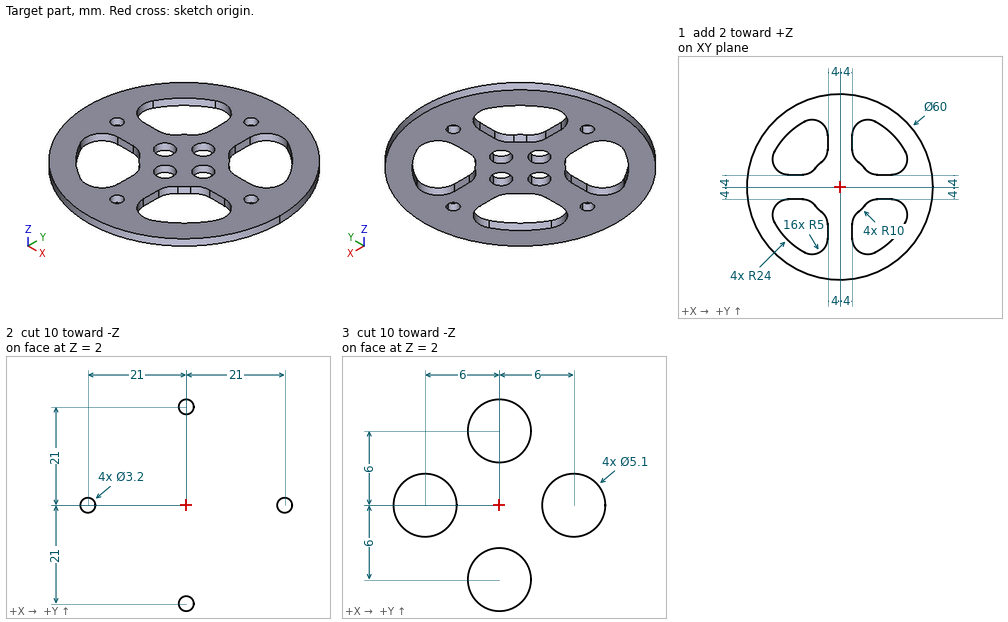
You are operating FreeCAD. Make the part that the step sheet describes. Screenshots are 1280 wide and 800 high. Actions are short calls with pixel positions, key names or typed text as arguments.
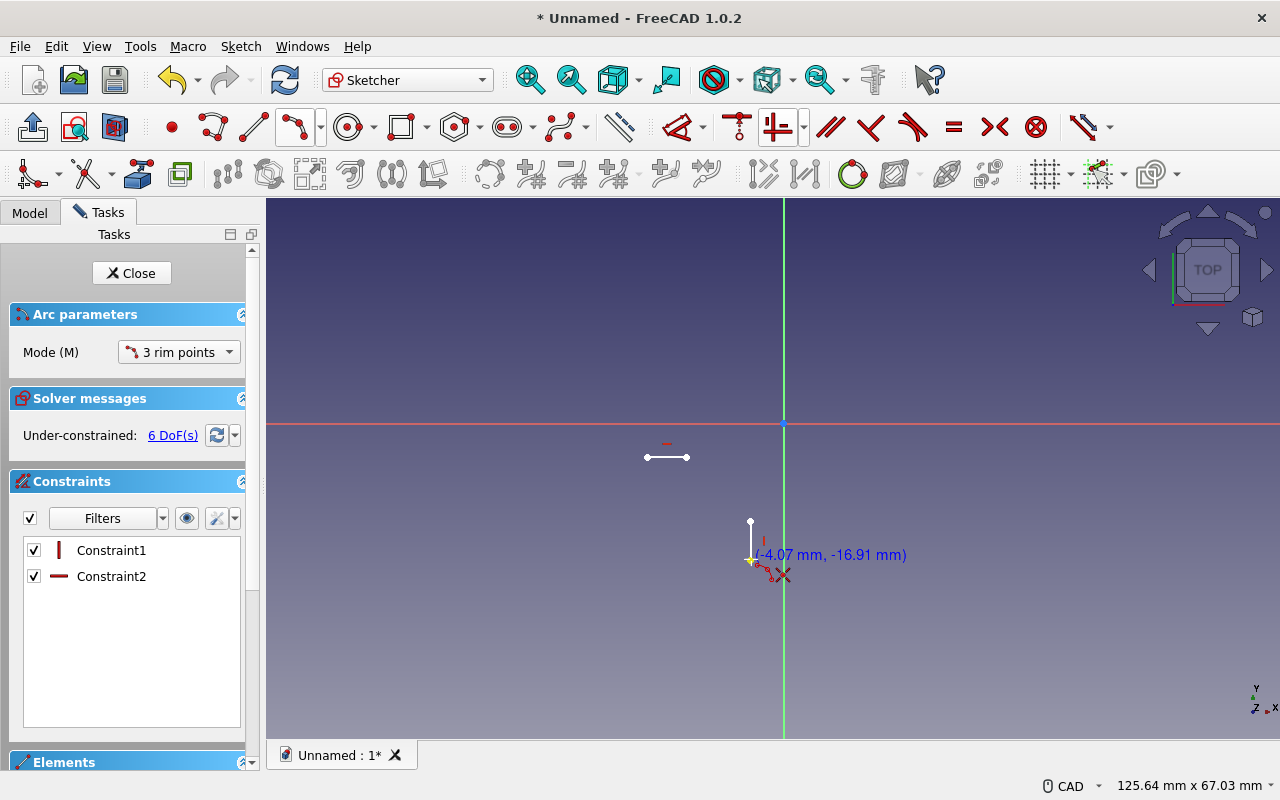
click(751, 560)
click(692, 594)
click(732, 593)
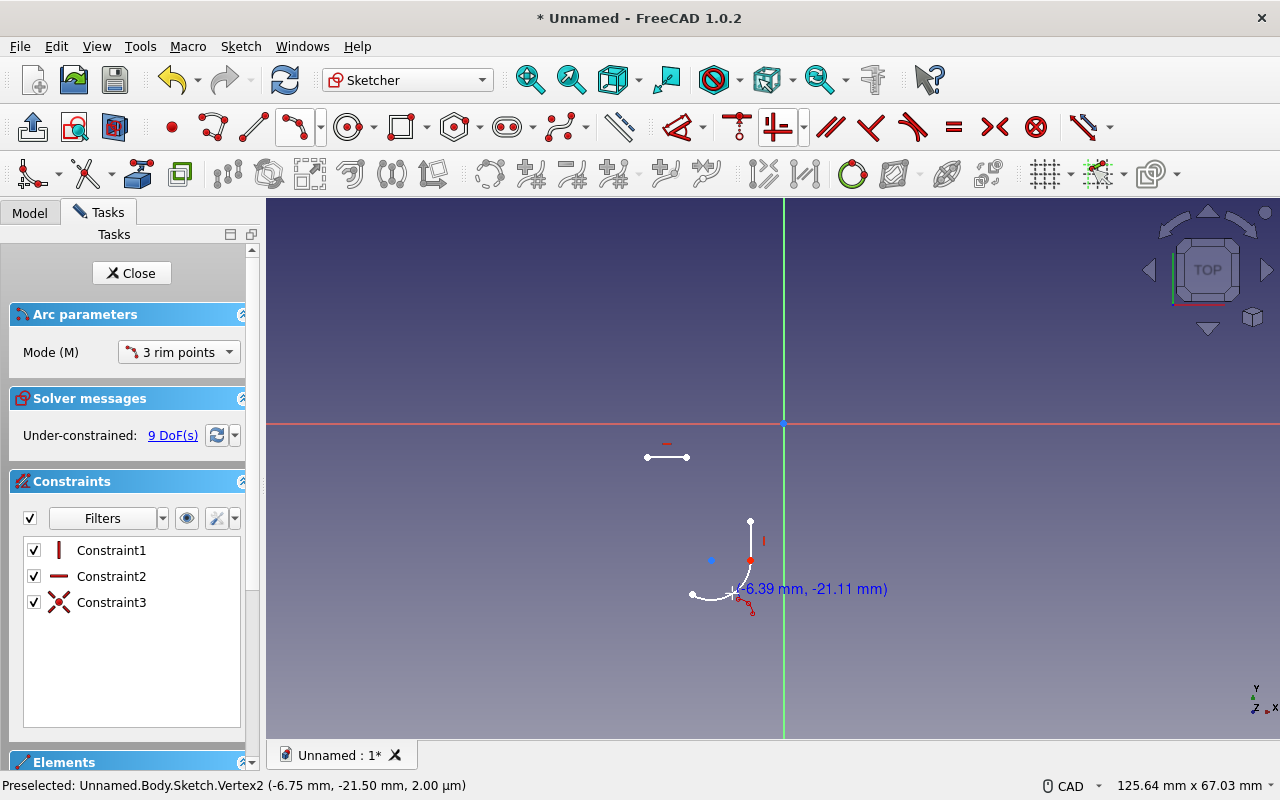
click(692, 595)
click(613, 515)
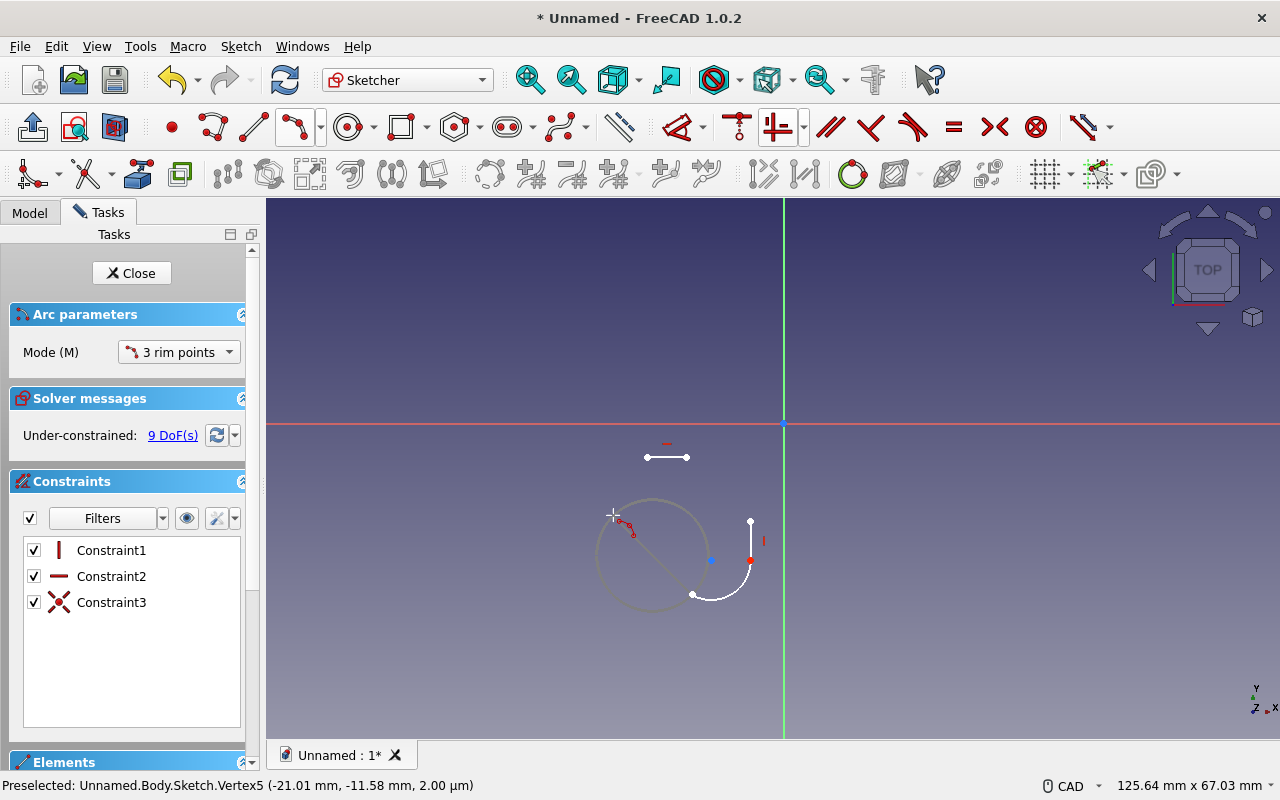
scroll(647, 561, up, 4)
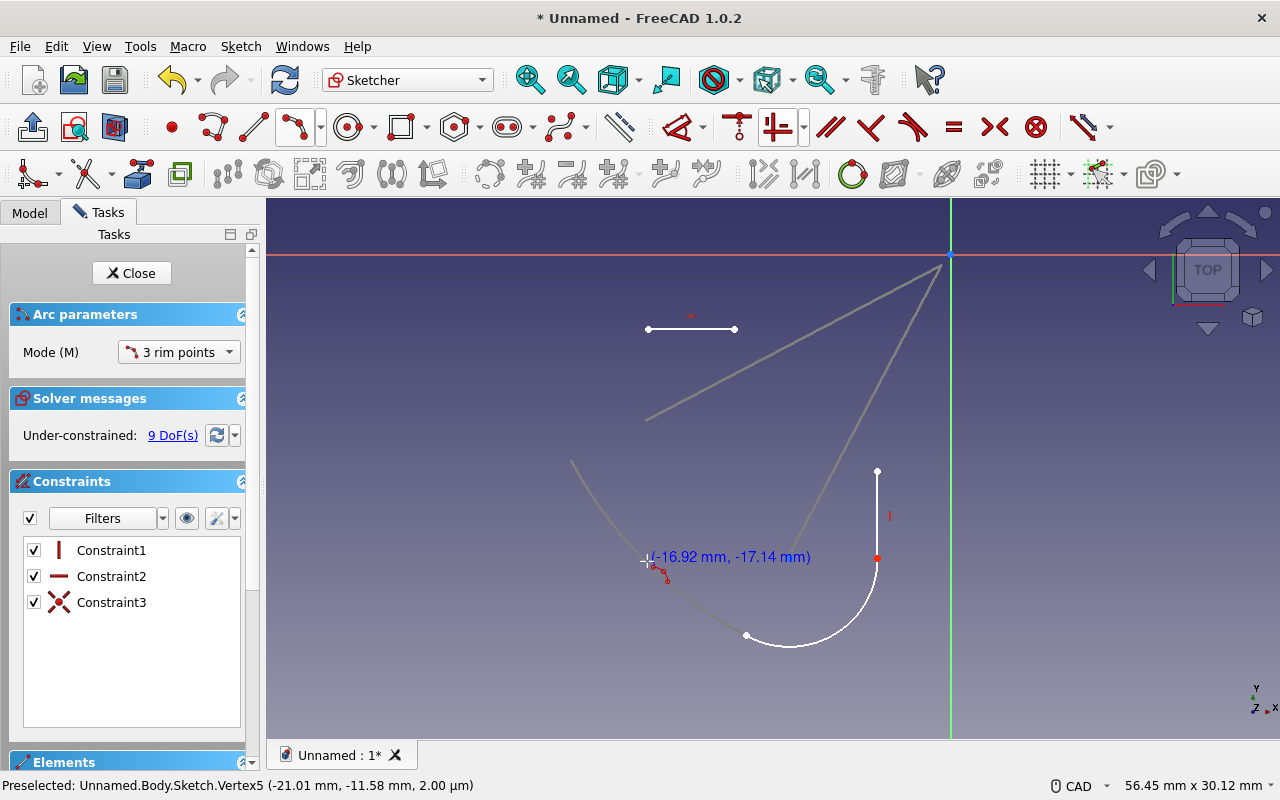
click(646, 559)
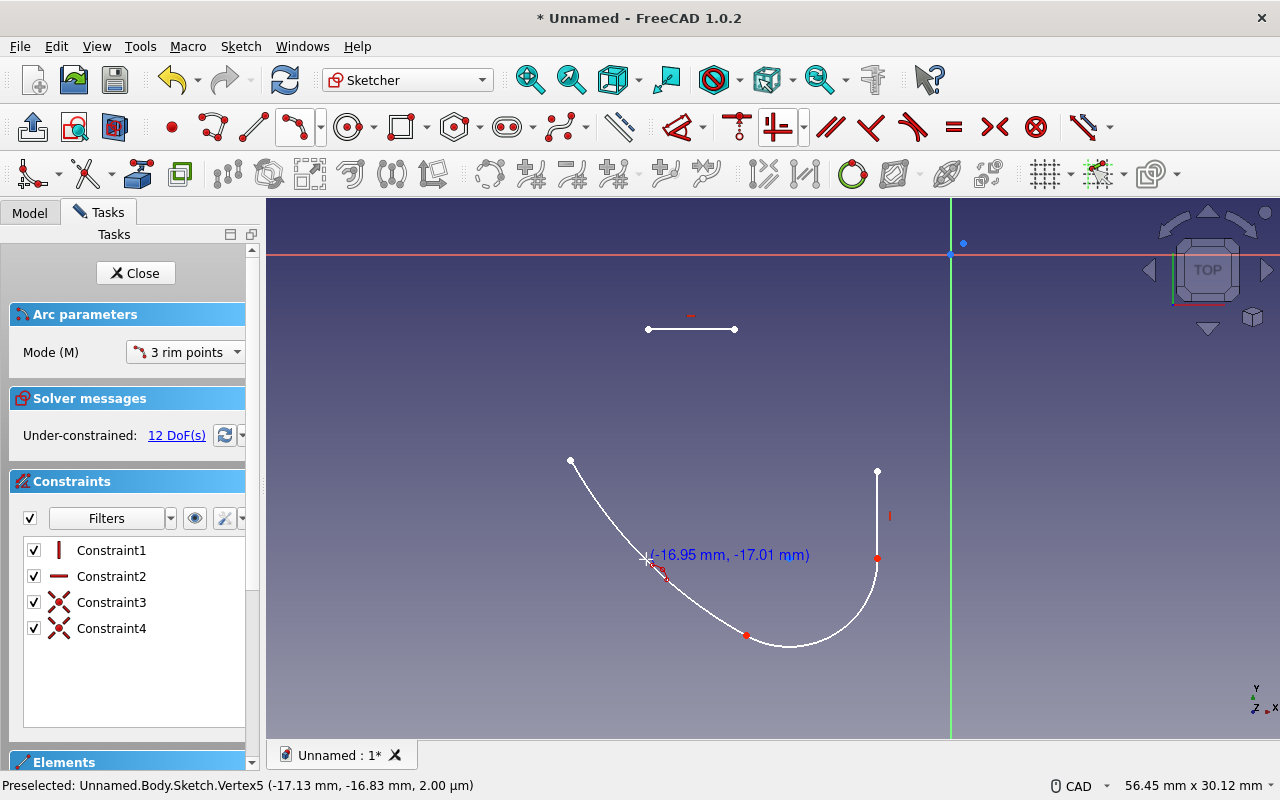
click(571, 460)
click(648, 329)
click(573, 370)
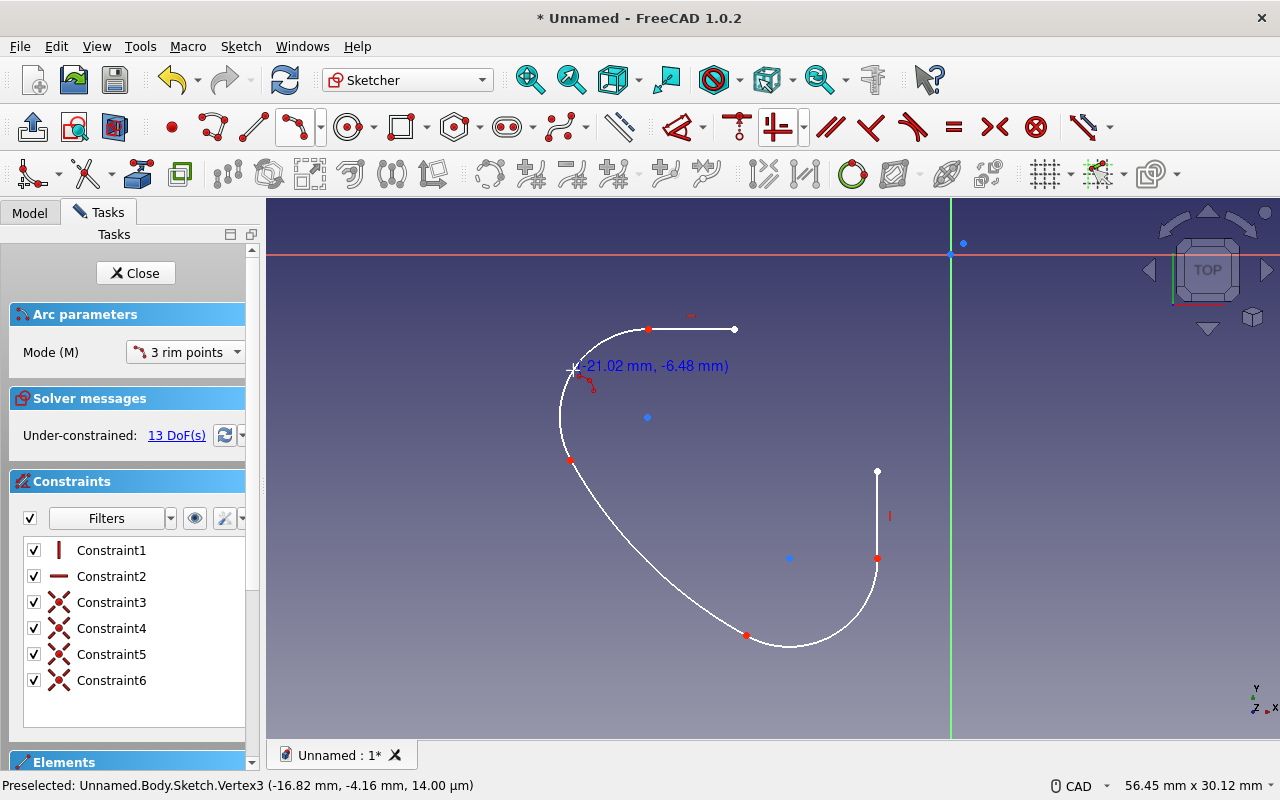
click(735, 329)
click(807, 362)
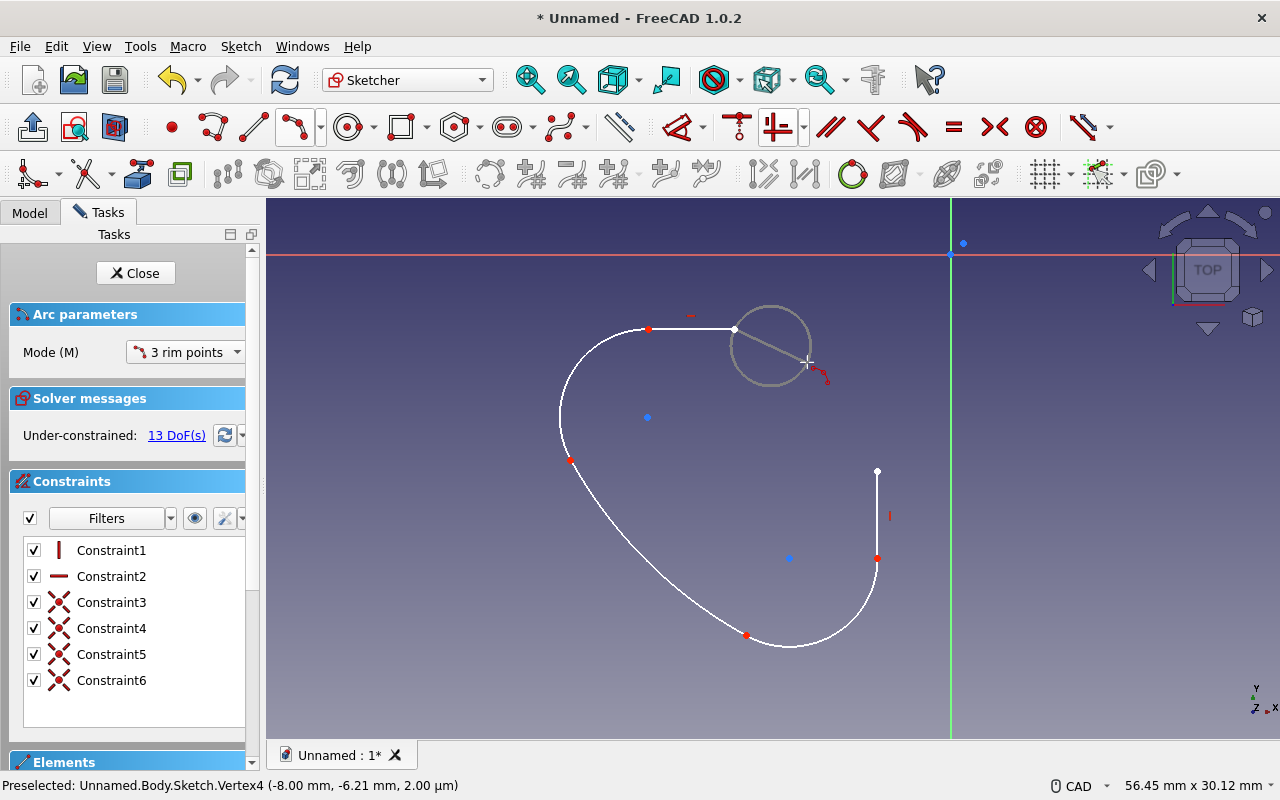
scroll(775, 336, up, 3)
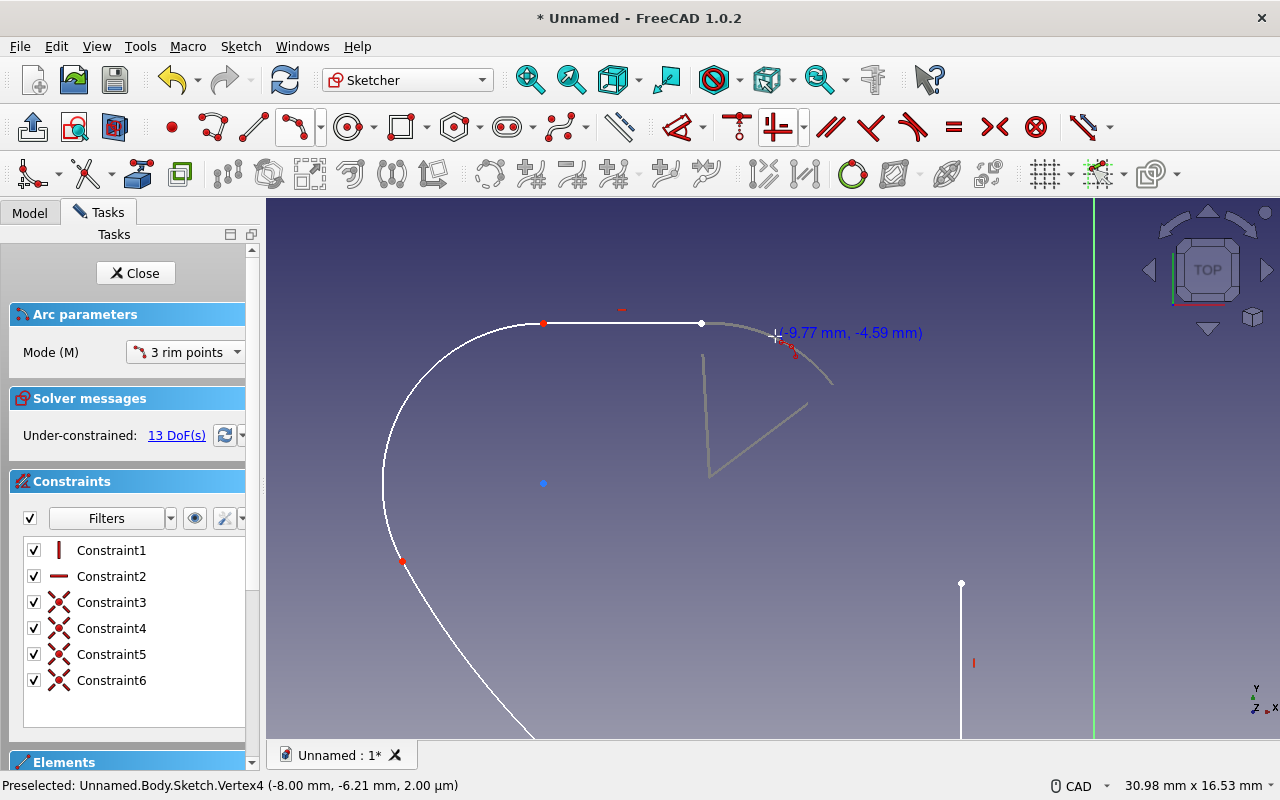
click(775, 336)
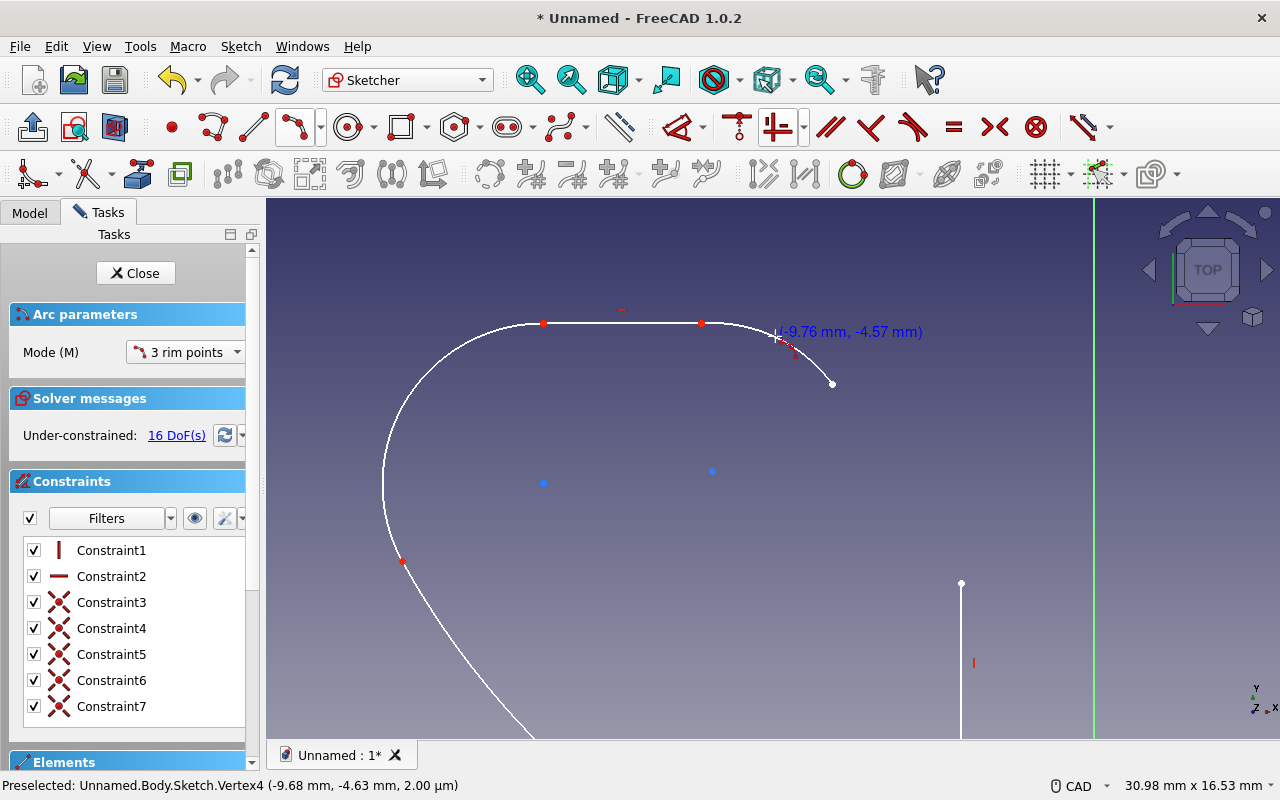
scroll(627, 524, down, 9)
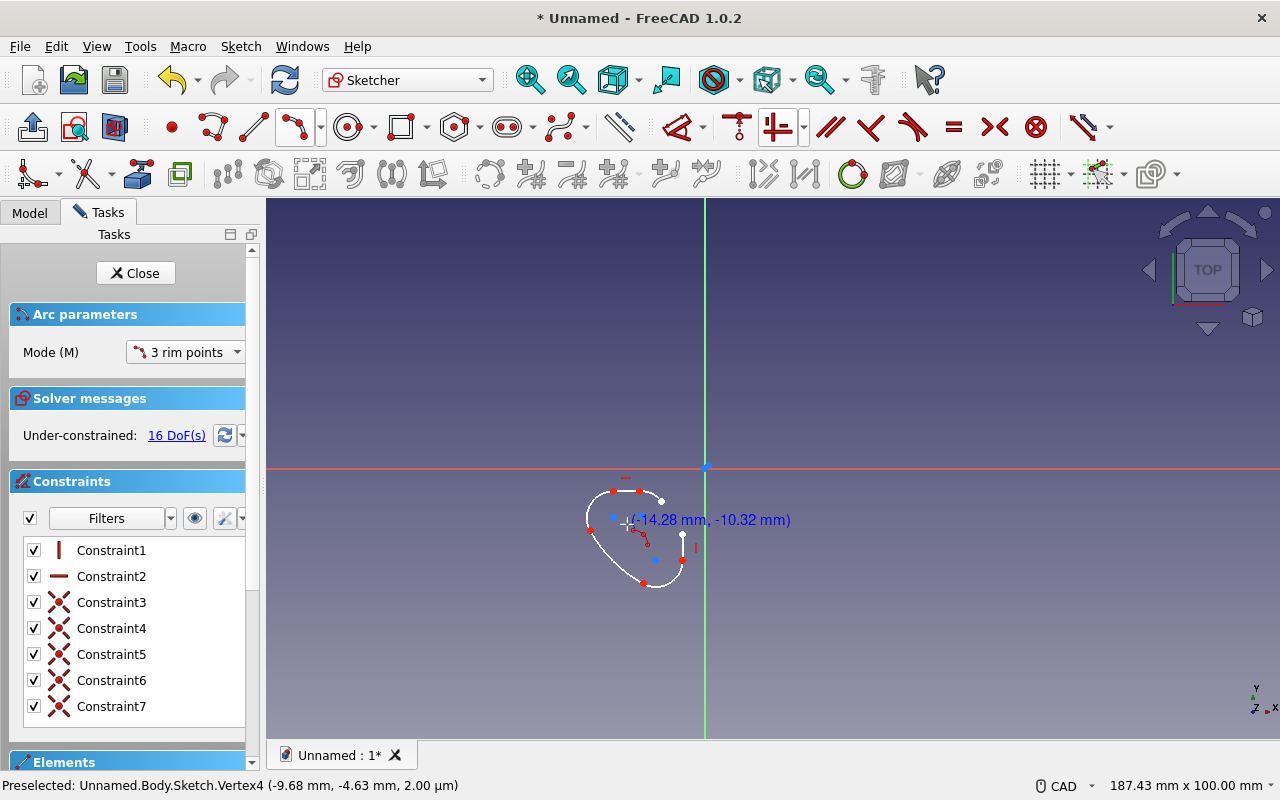
click(661, 502)
click(672, 512)